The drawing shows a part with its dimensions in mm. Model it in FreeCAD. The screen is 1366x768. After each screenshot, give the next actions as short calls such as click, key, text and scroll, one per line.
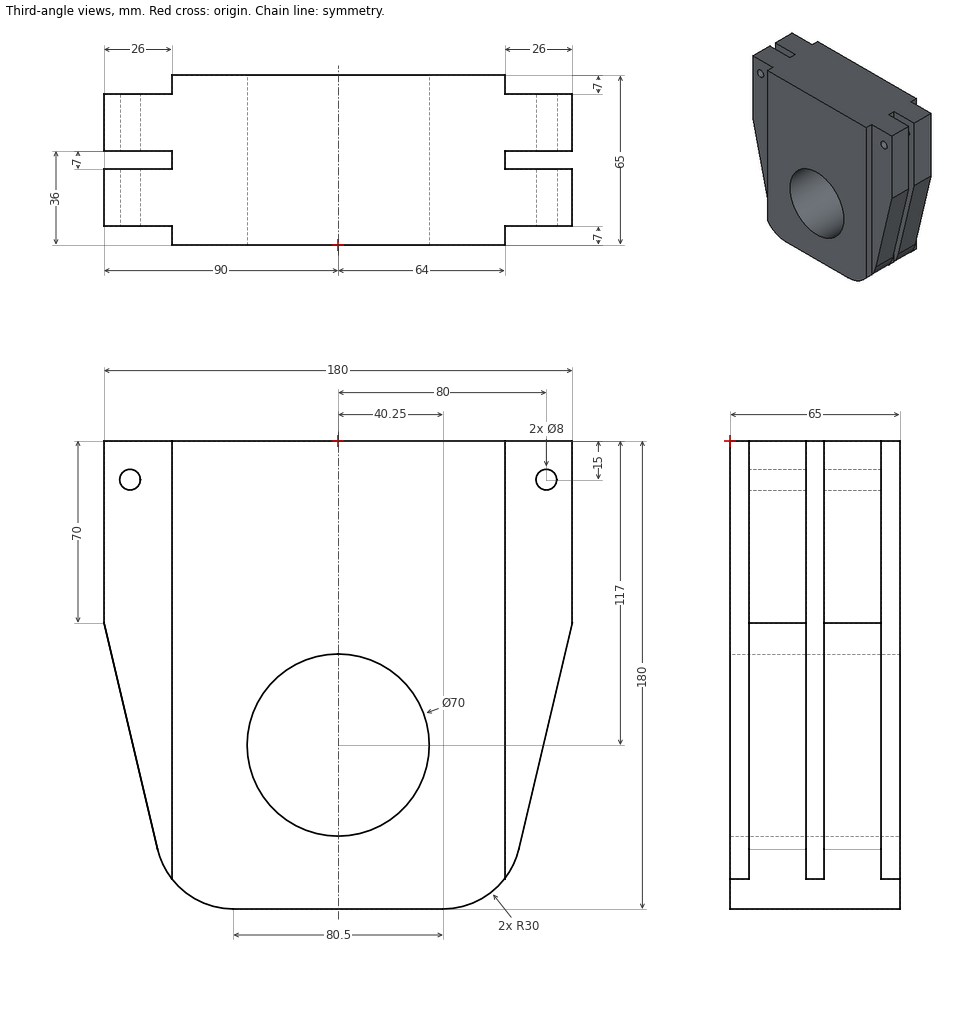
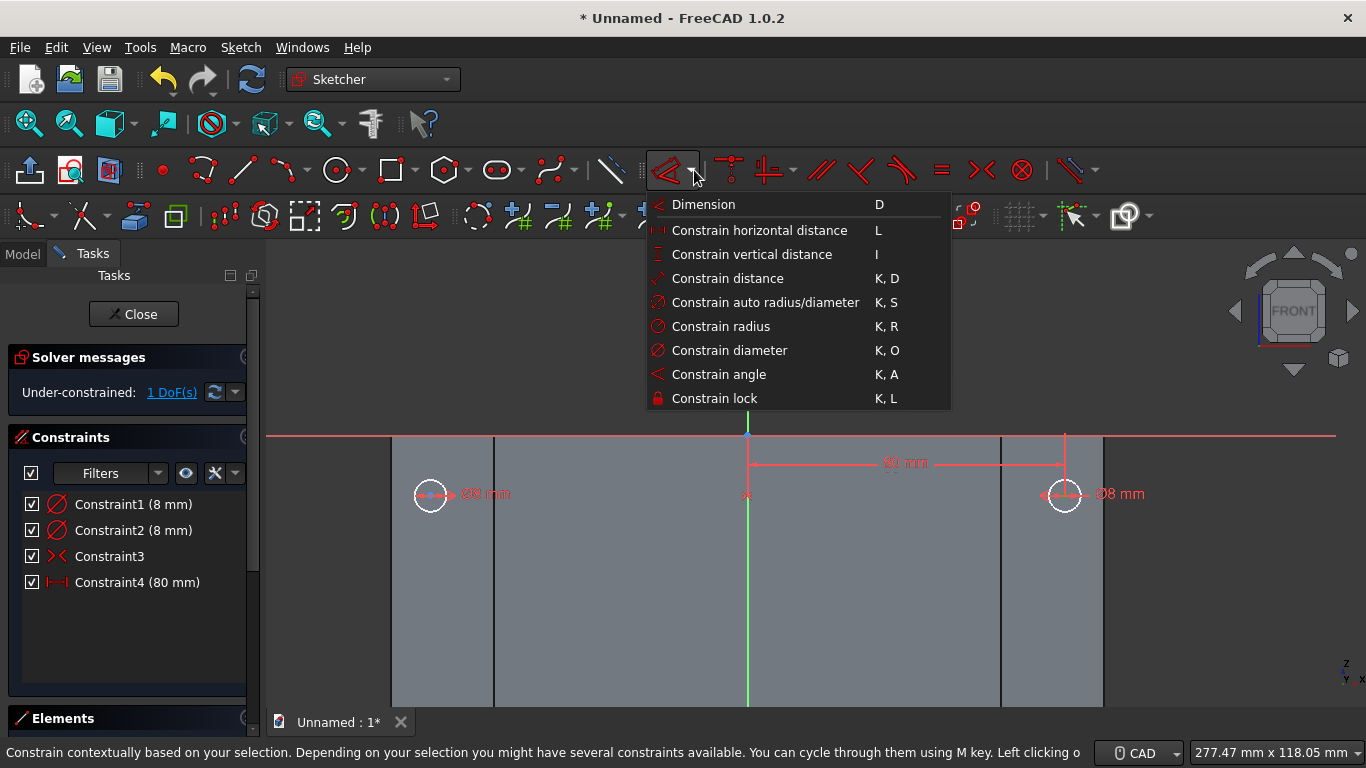
click(799, 254)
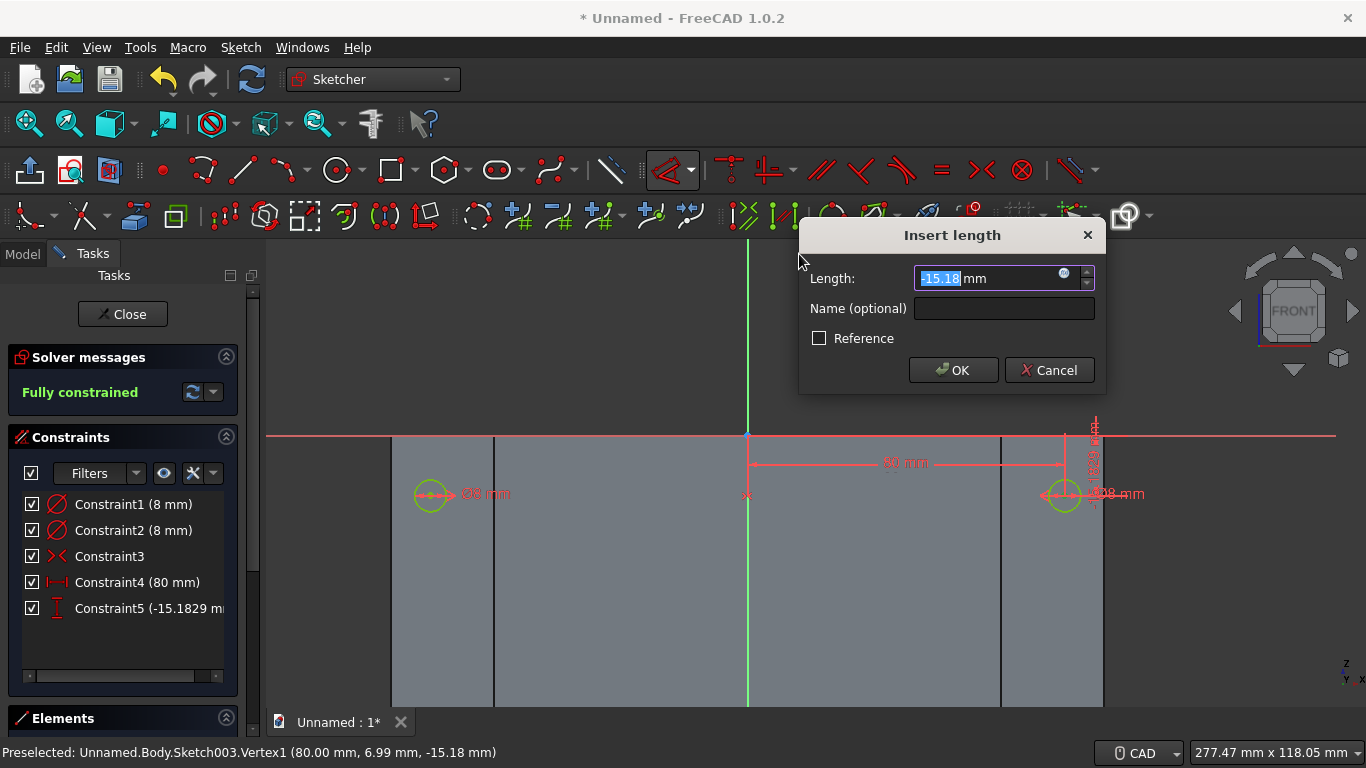
text(-15)
key(Return)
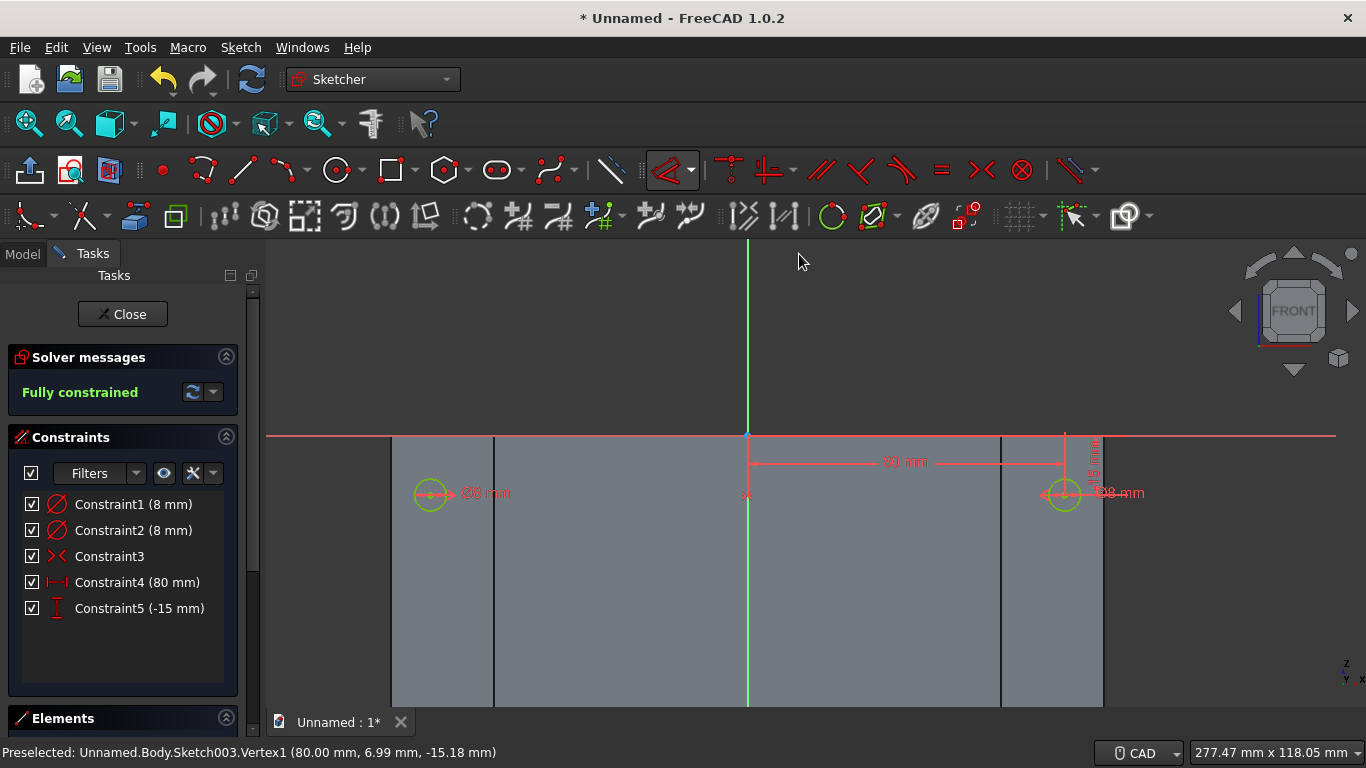
click(123, 314)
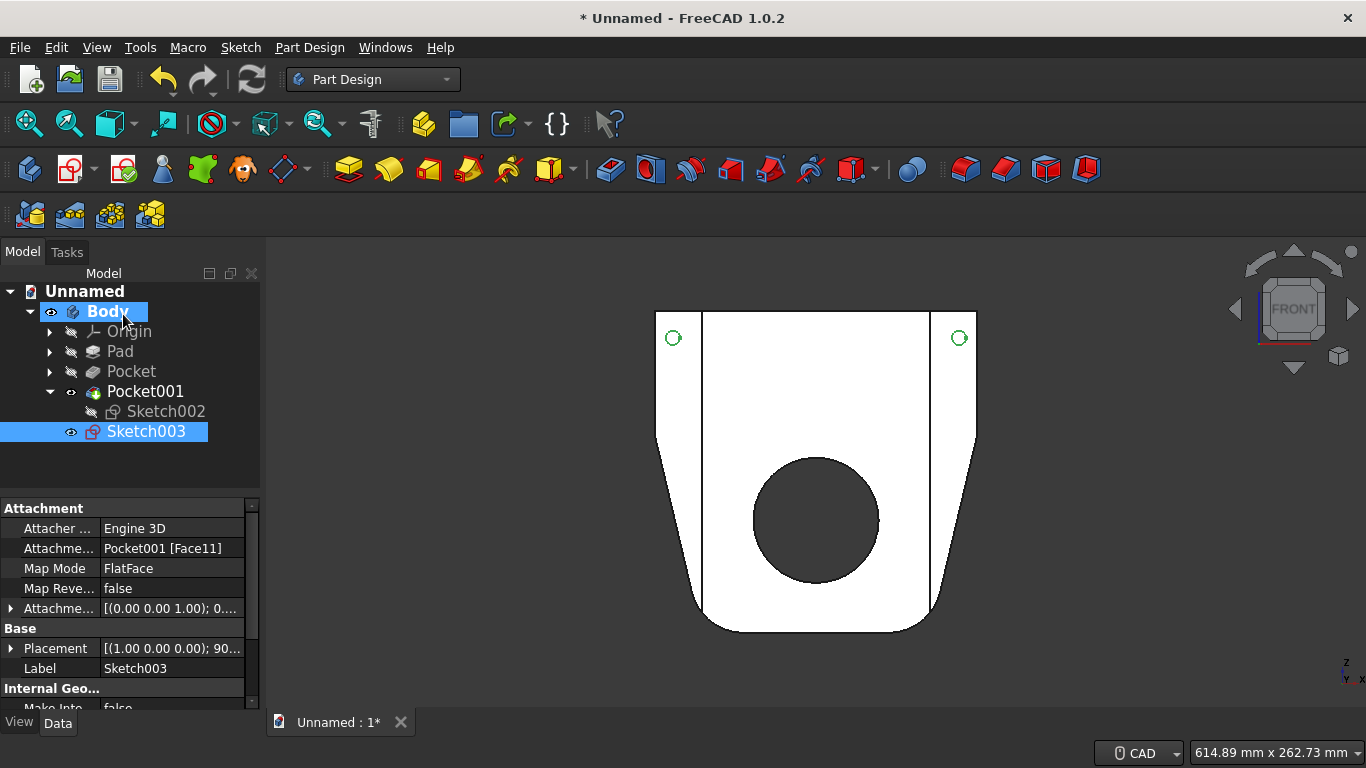
click(612, 170)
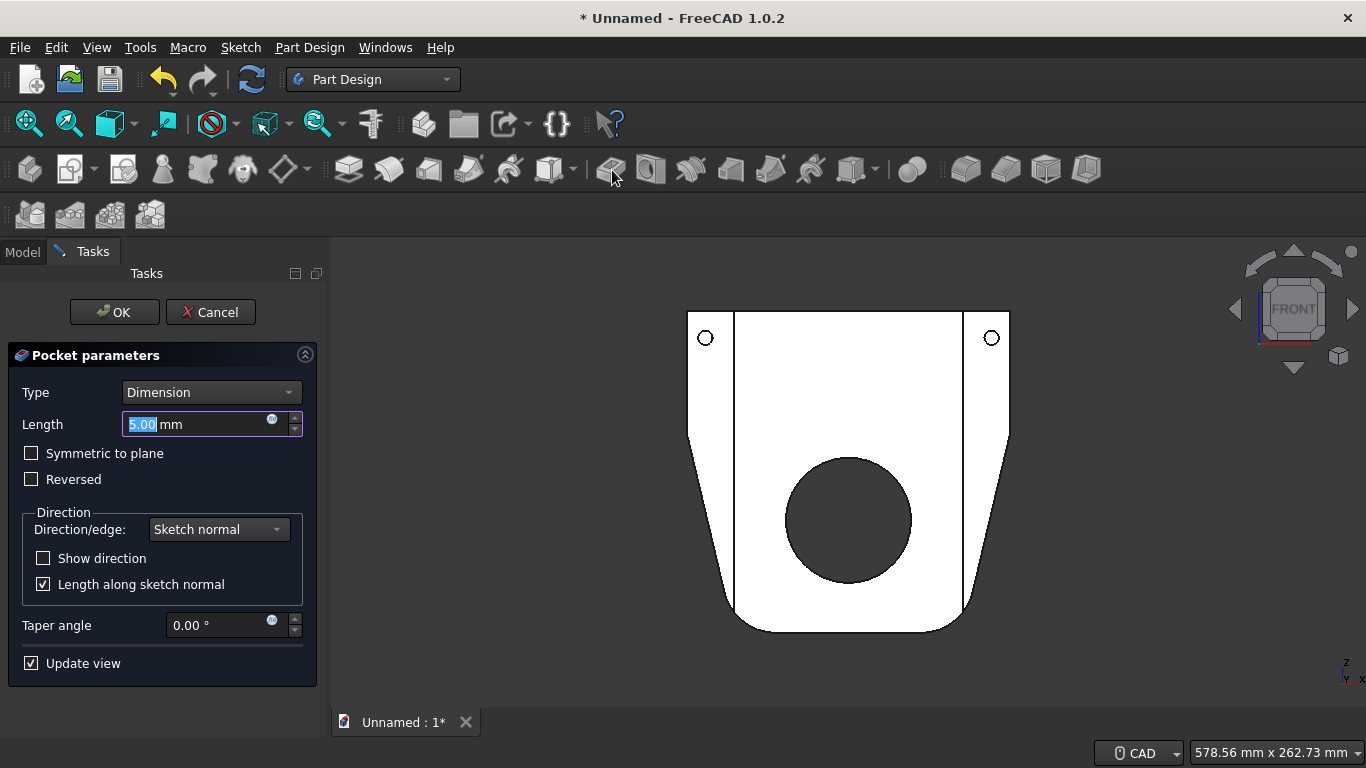
click(212, 392)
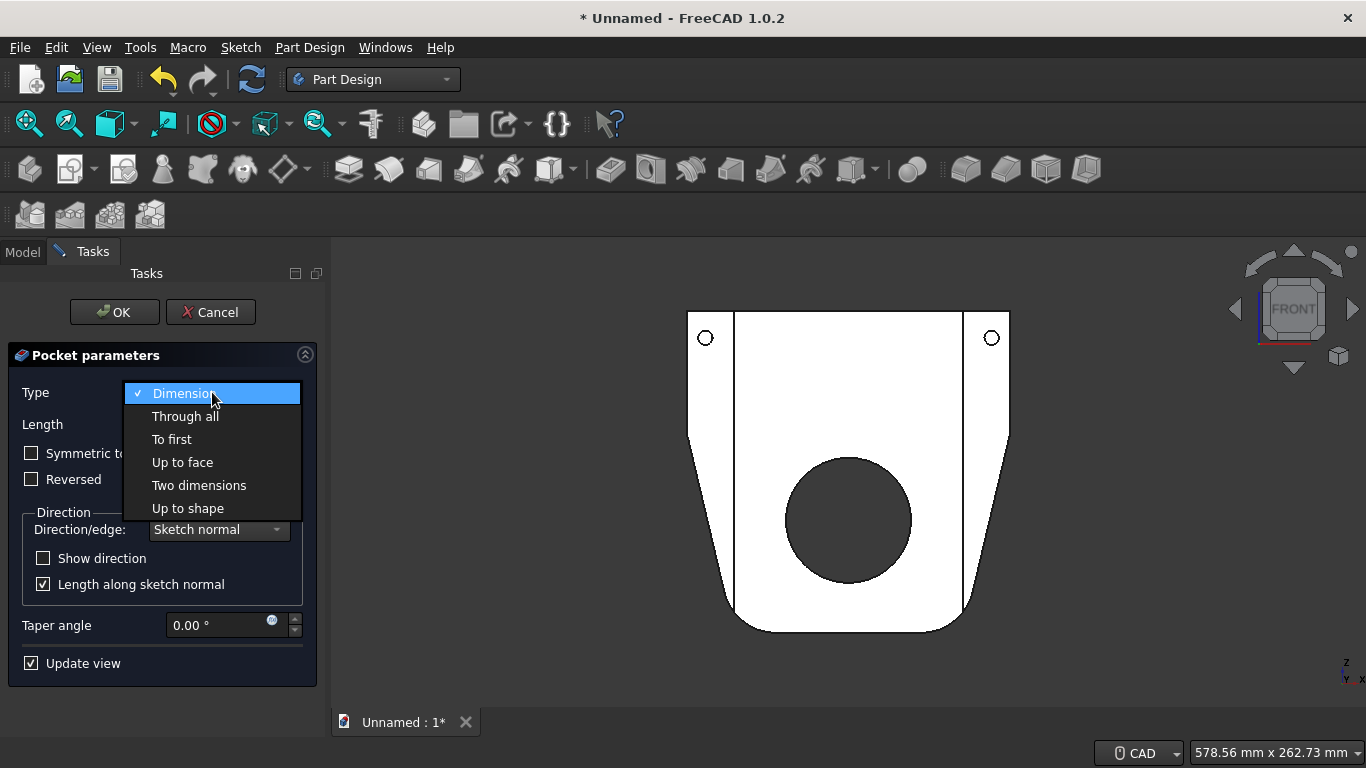
click(212, 416)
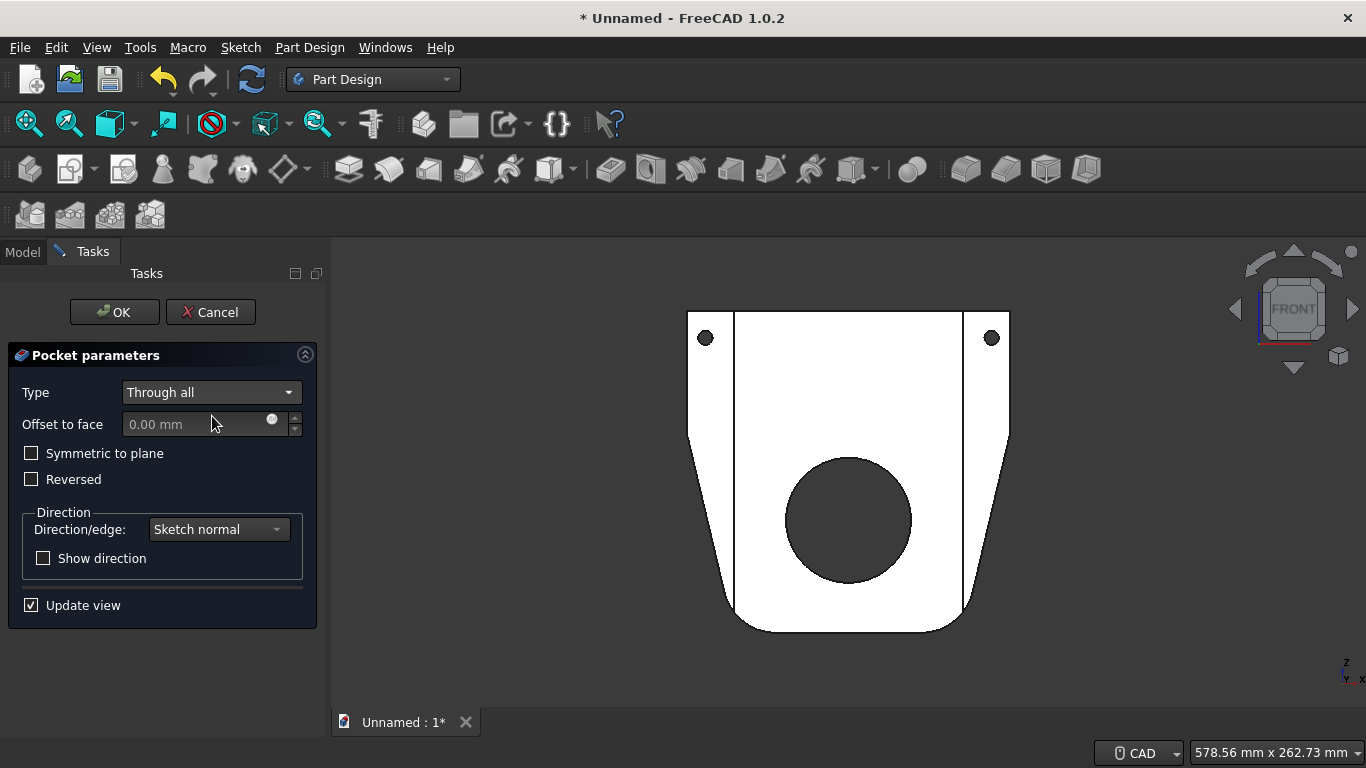
click(115, 312)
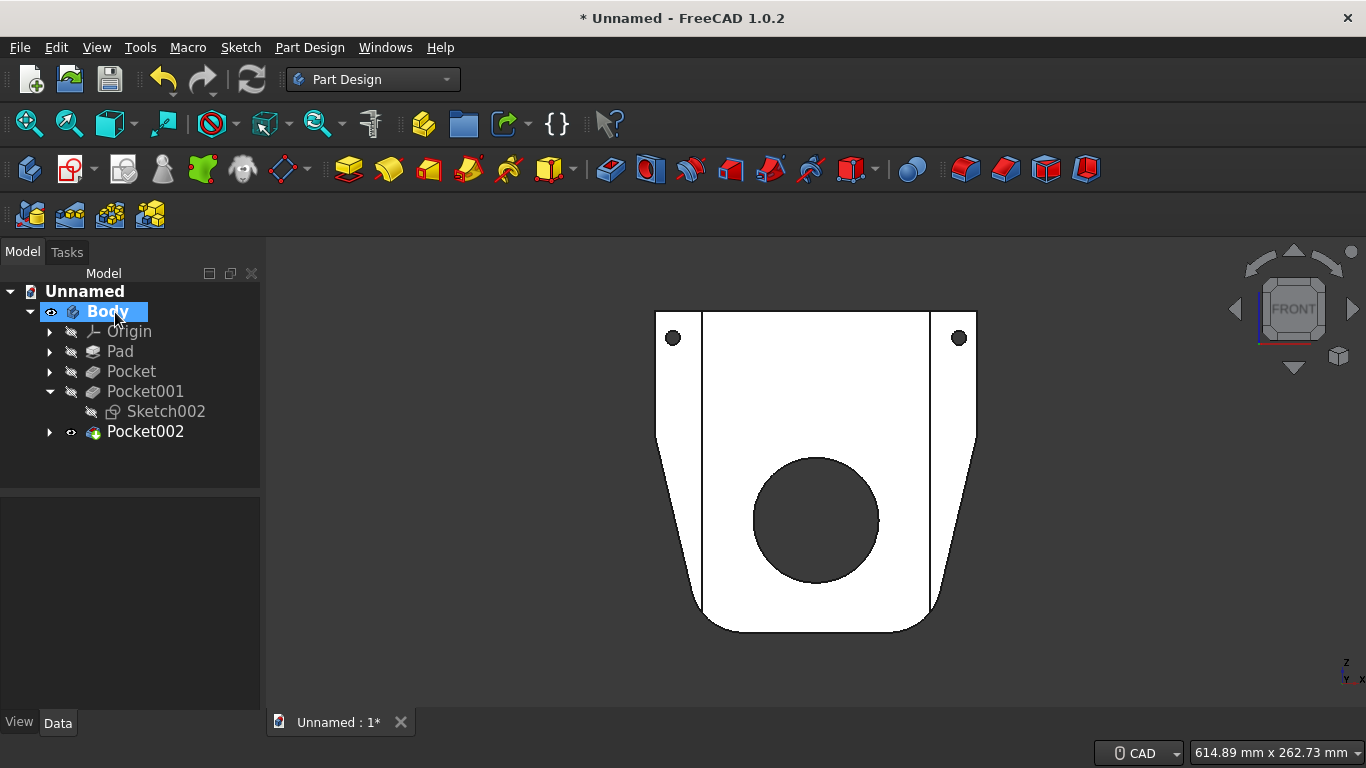
click(70, 170)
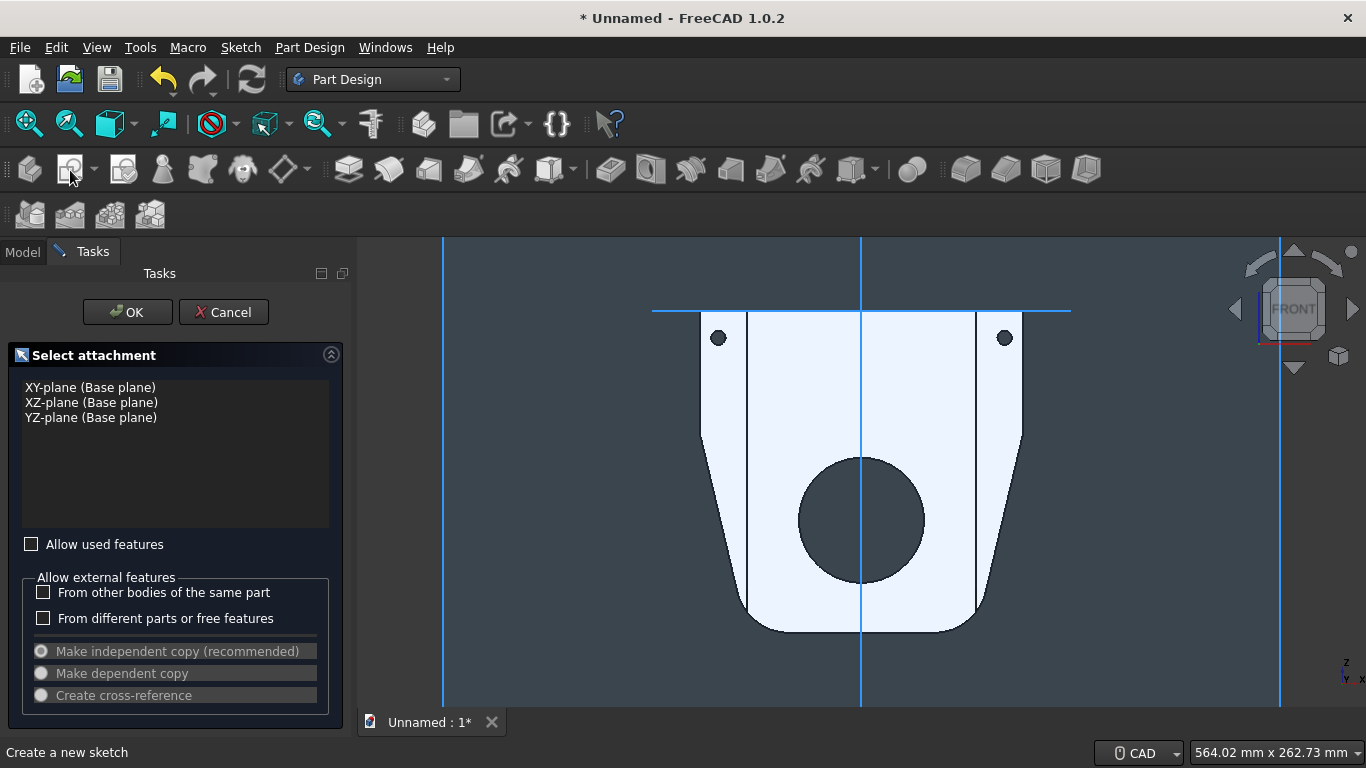
click(82, 388)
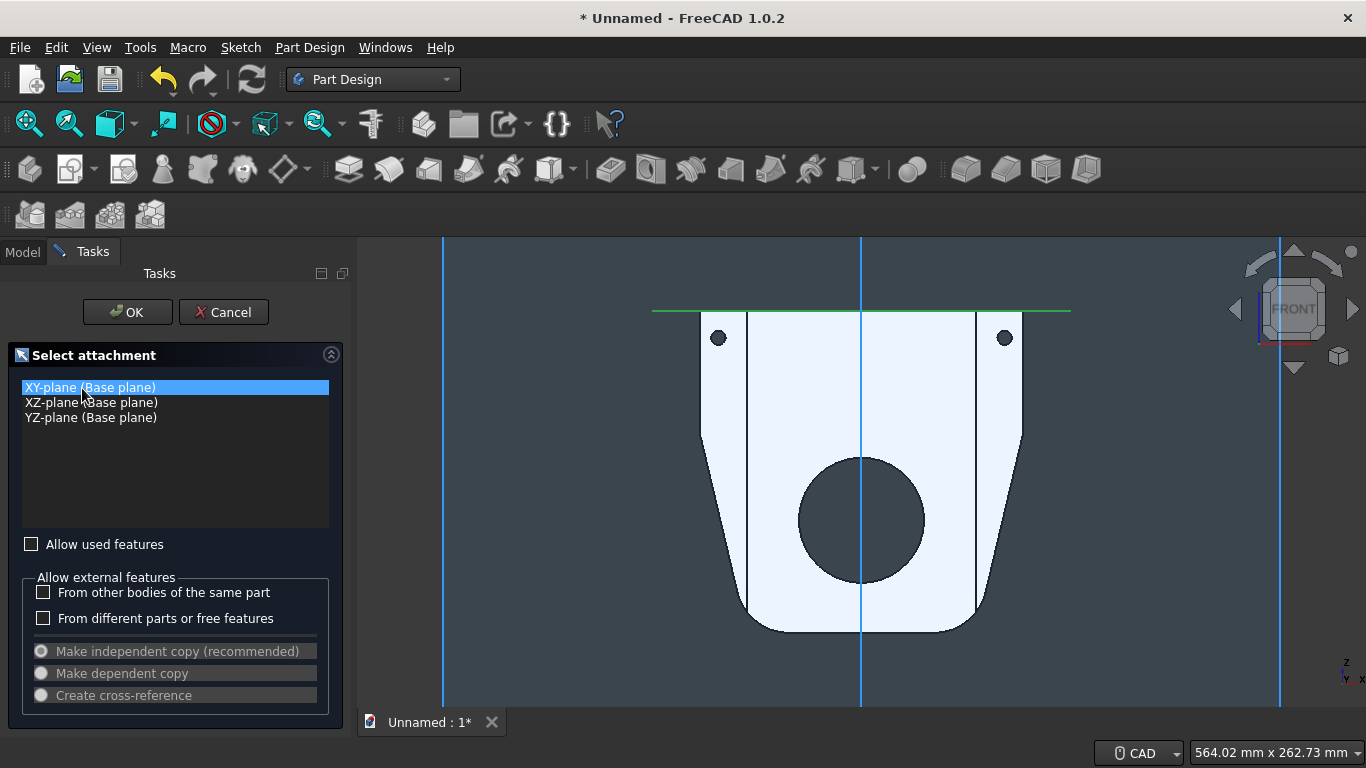
click(128, 312)